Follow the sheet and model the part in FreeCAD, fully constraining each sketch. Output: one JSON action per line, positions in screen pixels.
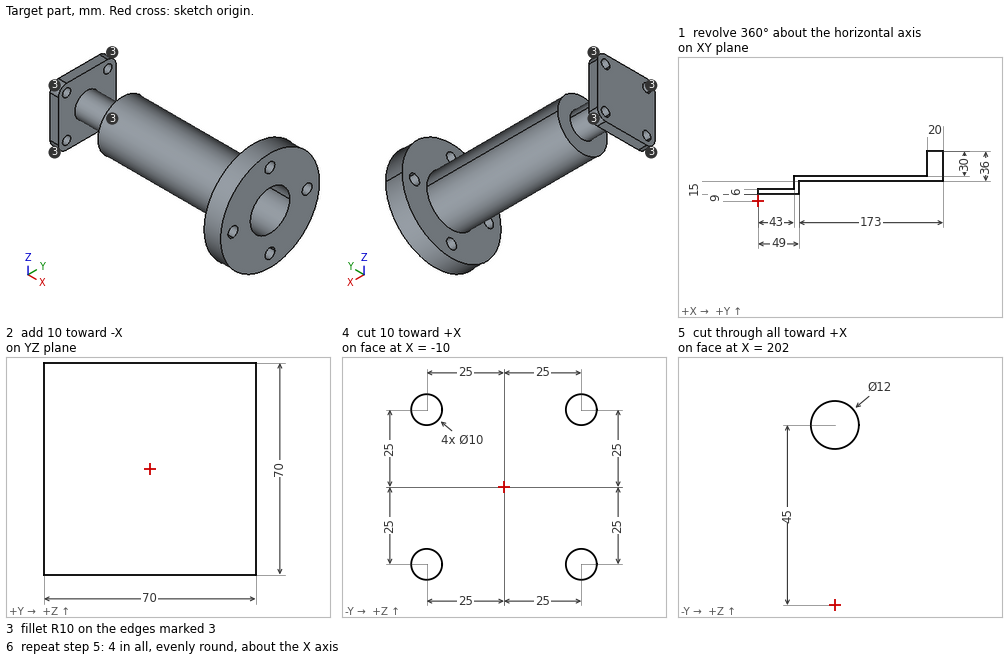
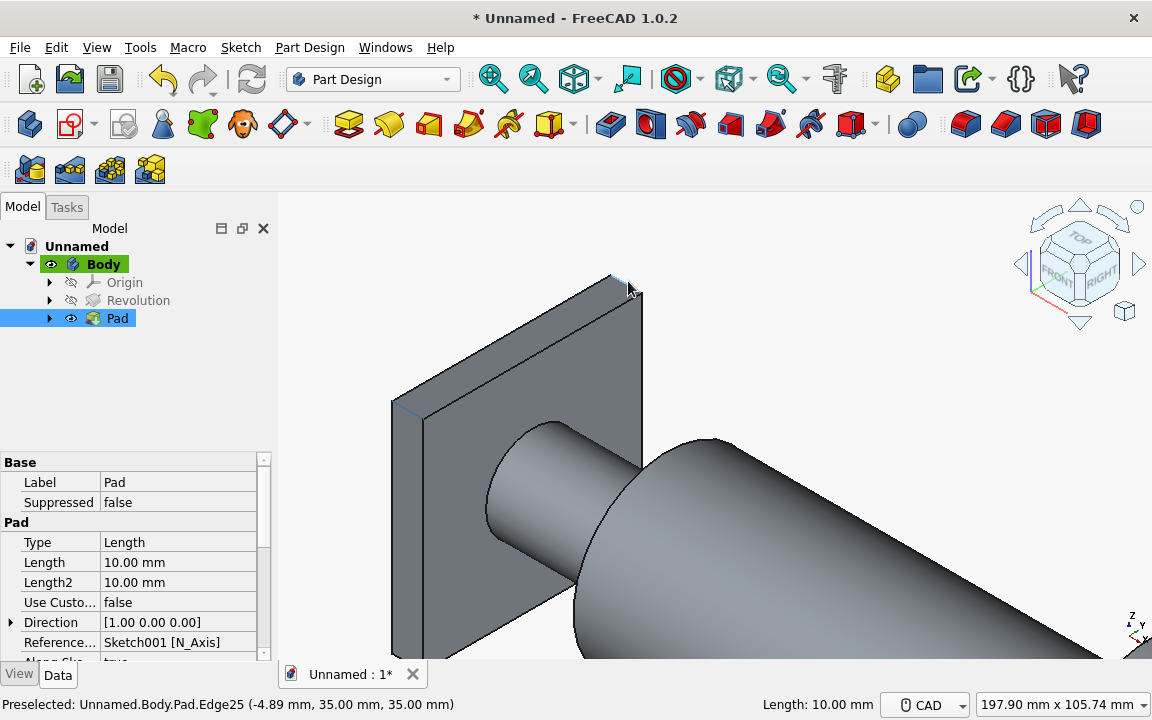
{"action": "left_click", "coordinate": [494, 80]}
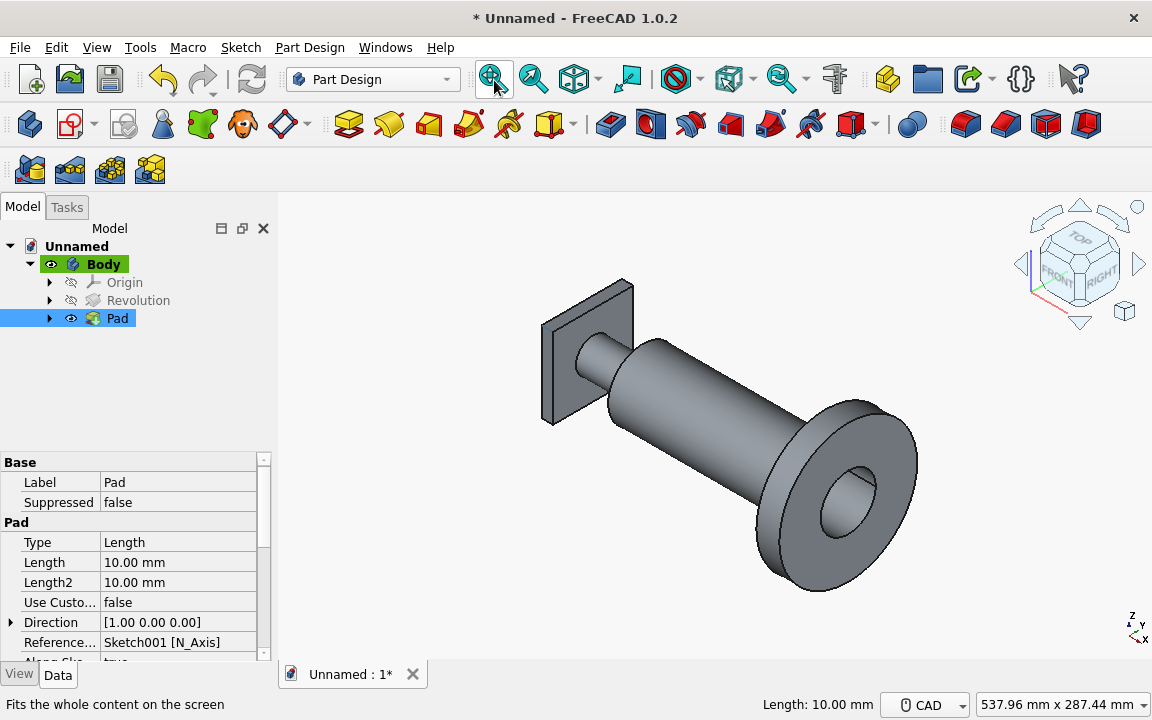
{"action": "key", "text": "2"}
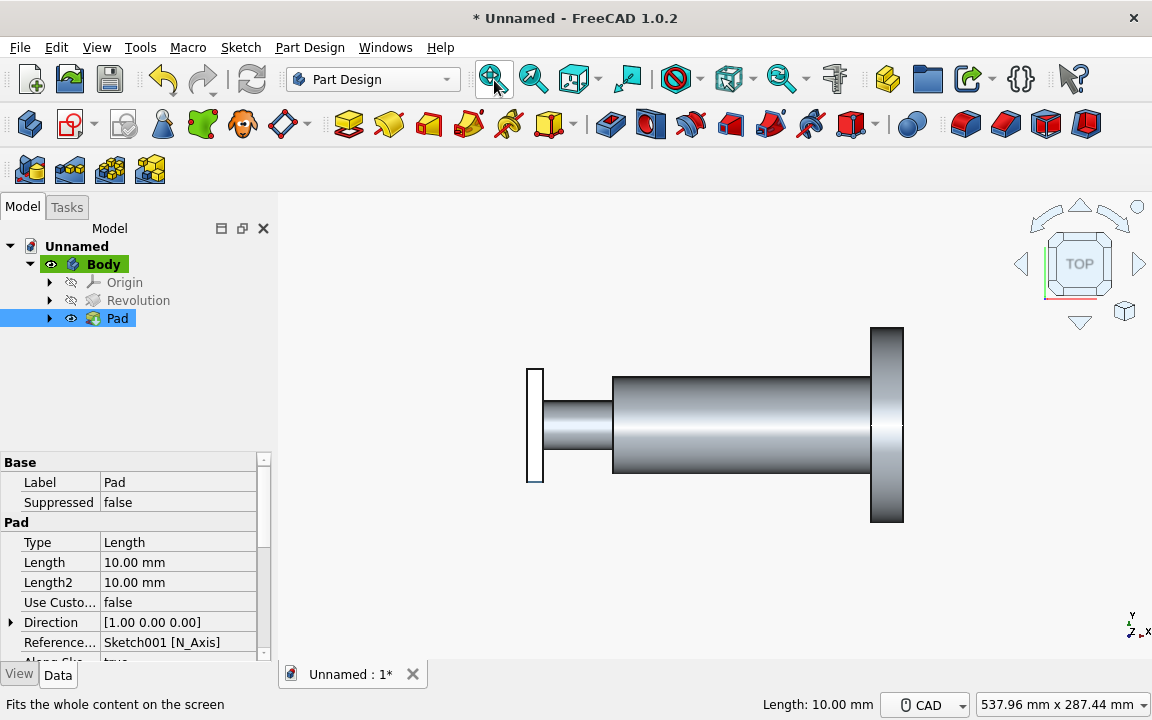
{"action": "left_click", "coordinate": [494, 80]}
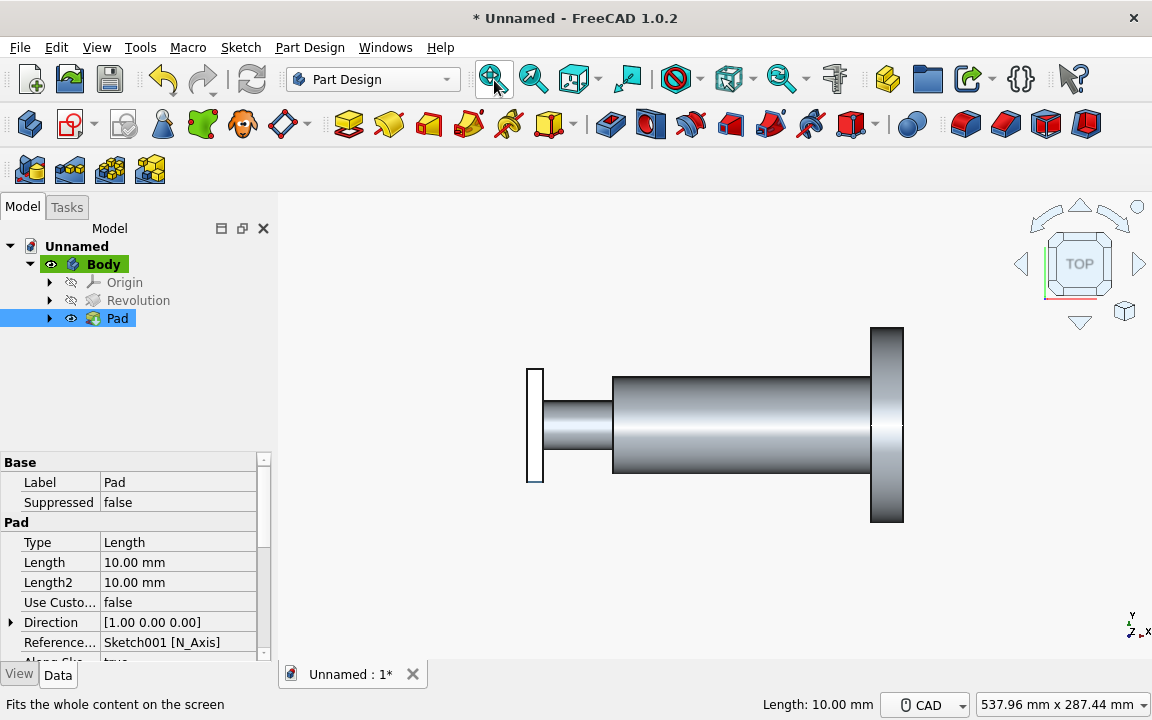
{"action": "left_click", "coordinate": [535, 368], "text": "ctrl"}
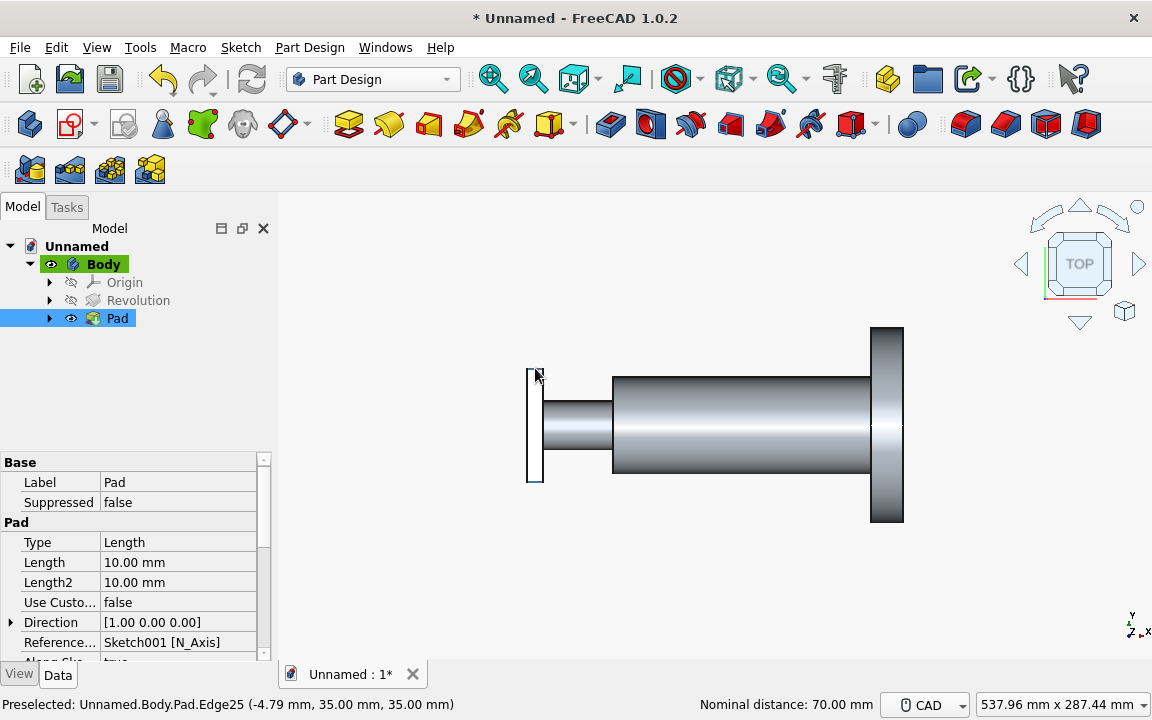
{"action": "scroll", "coordinate": [535, 368], "scroll_direction": "up", "scroll_amount": 5}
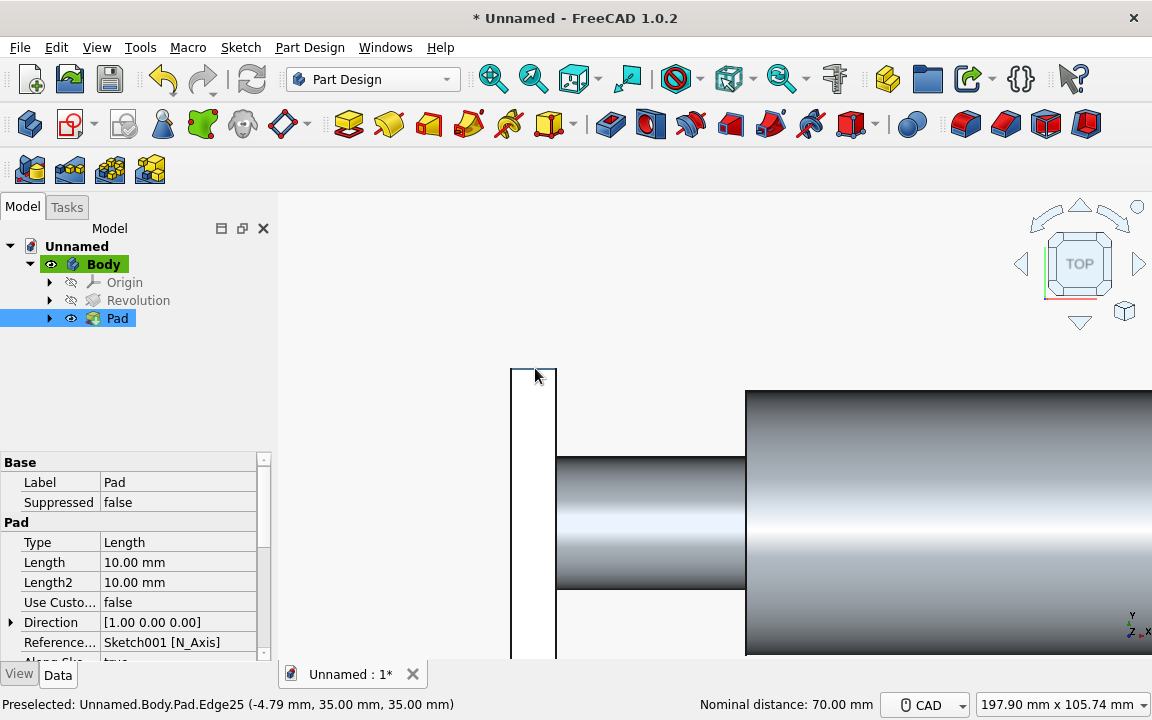
{"action": "key", "text": "v f"}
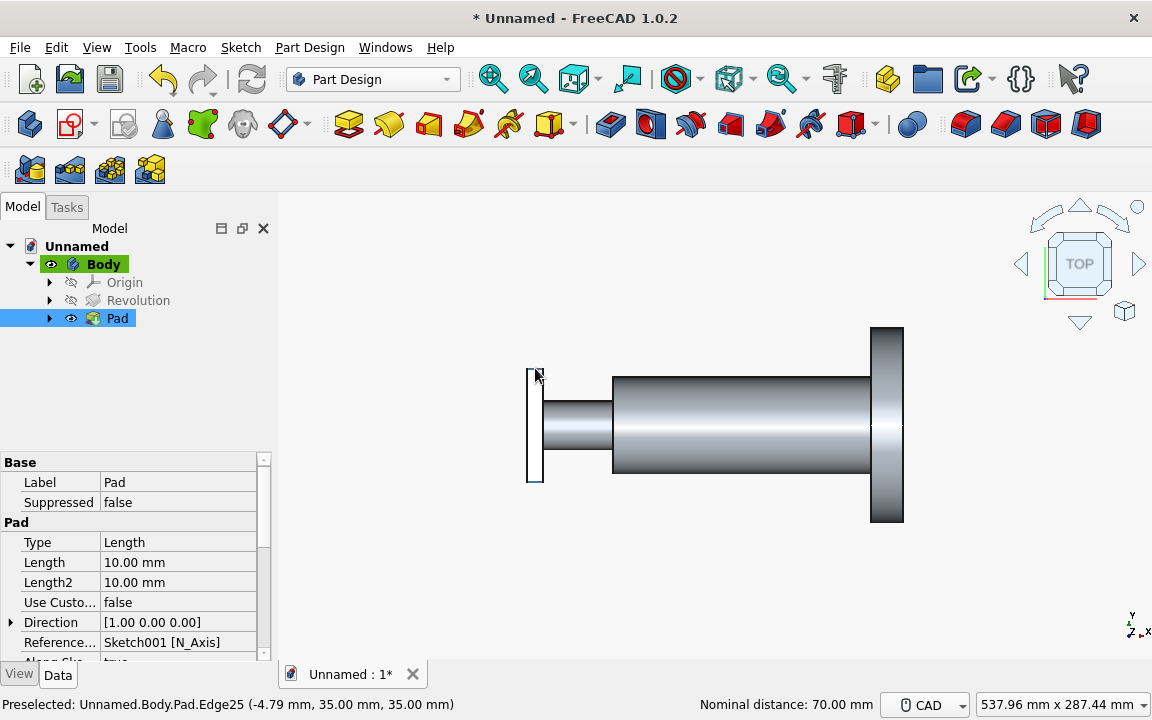
{"action": "key", "text": "1"}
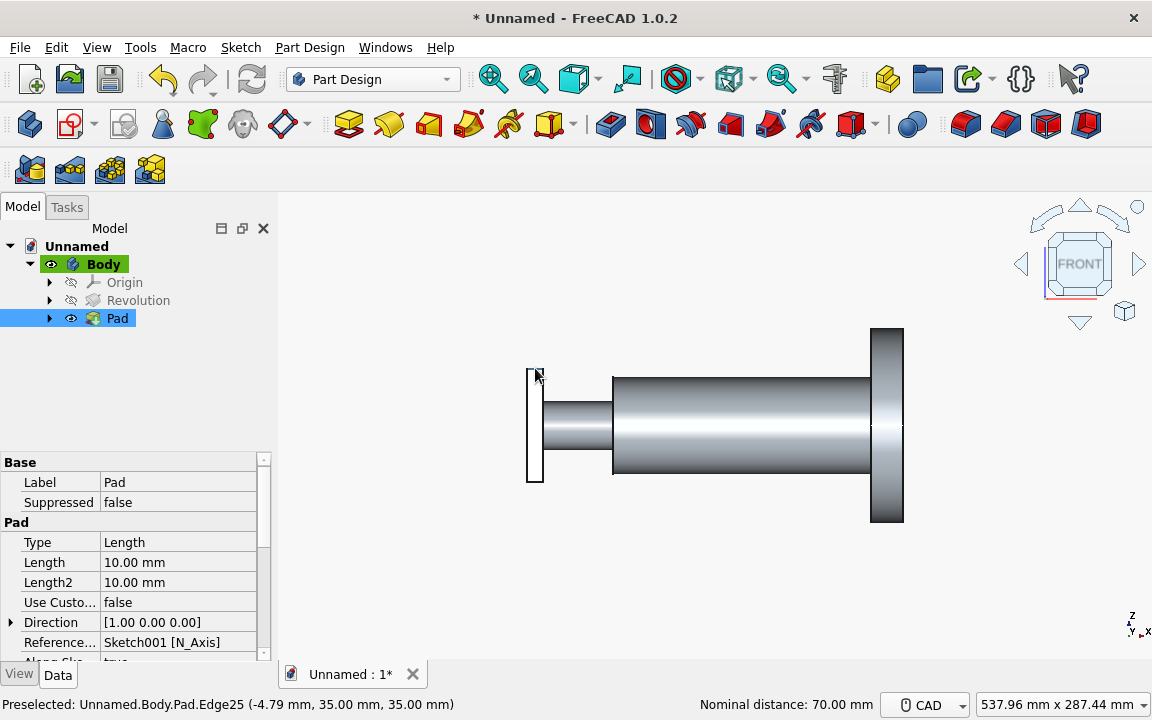
{"action": "key", "text": "v f"}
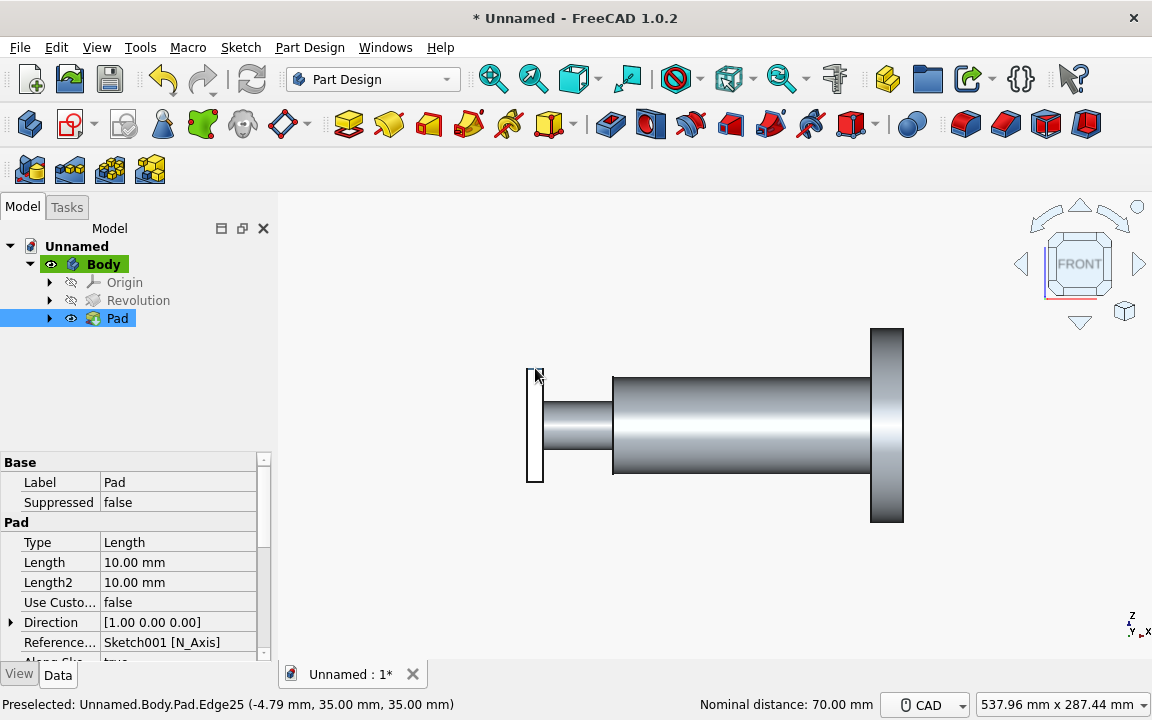
{"action": "left_click", "coordinate": [535, 481], "text": "ctrl"}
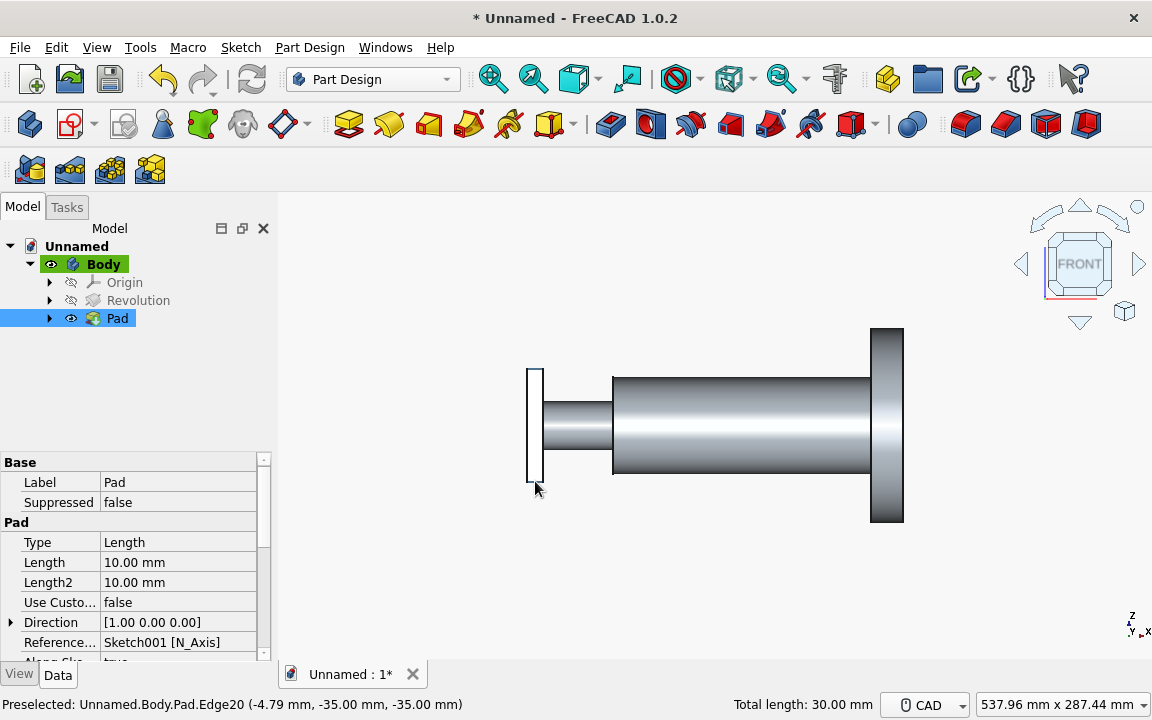
{"action": "scroll", "coordinate": [535, 481], "scroll_direction": "up", "scroll_amount": 5}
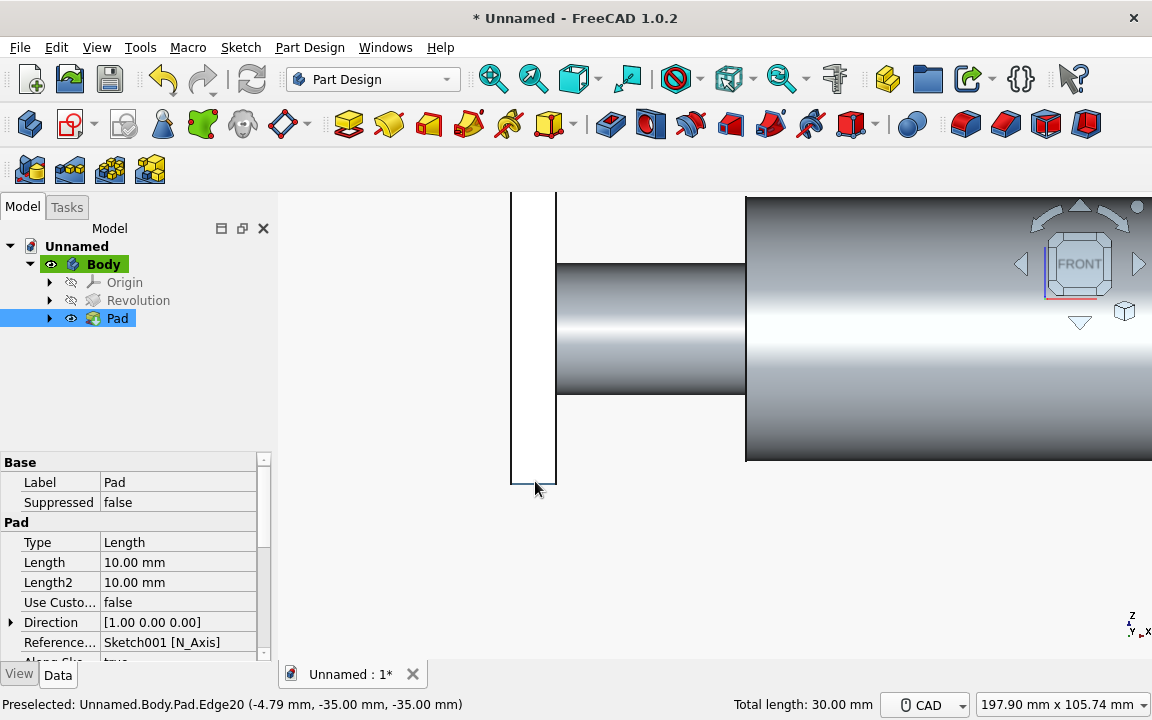
{"action": "left_click", "coordinate": [494, 80]}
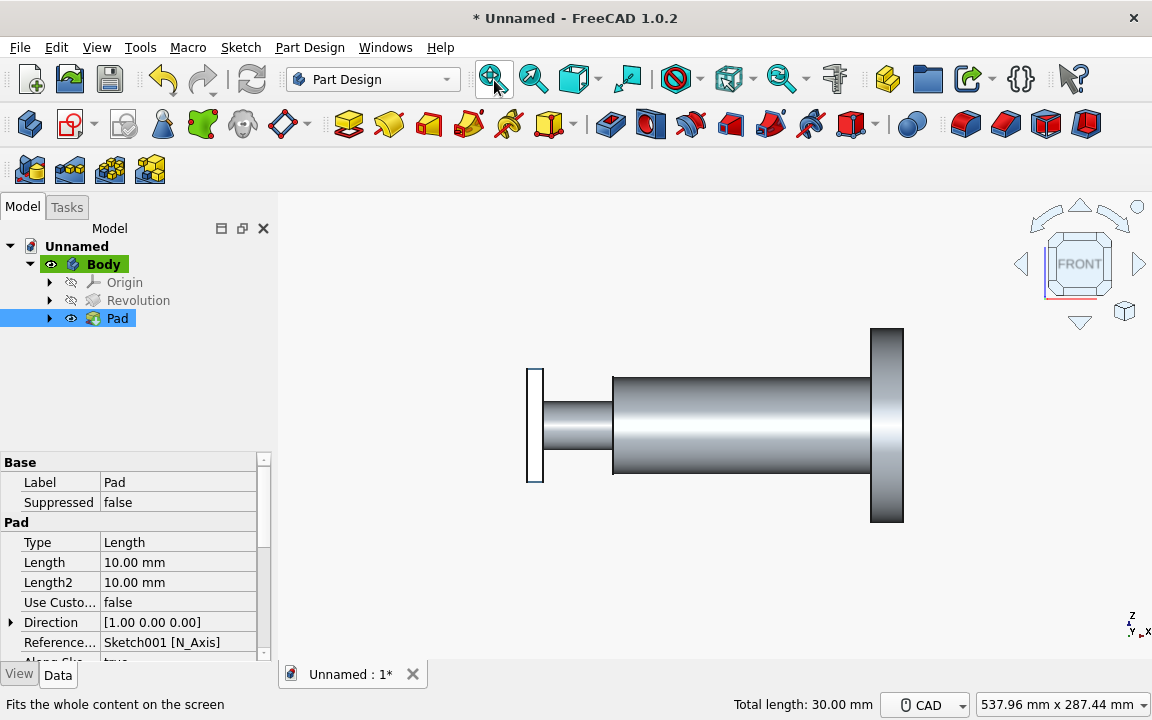
{"action": "key", "text": "3"}